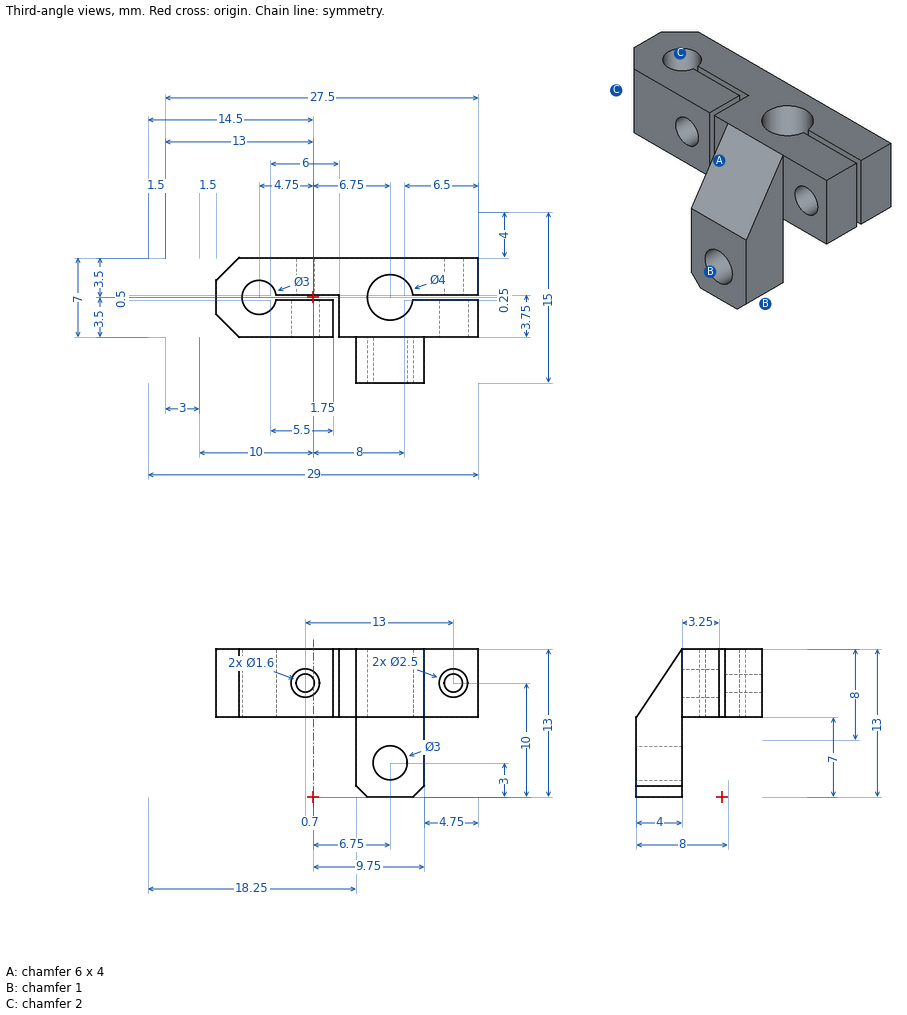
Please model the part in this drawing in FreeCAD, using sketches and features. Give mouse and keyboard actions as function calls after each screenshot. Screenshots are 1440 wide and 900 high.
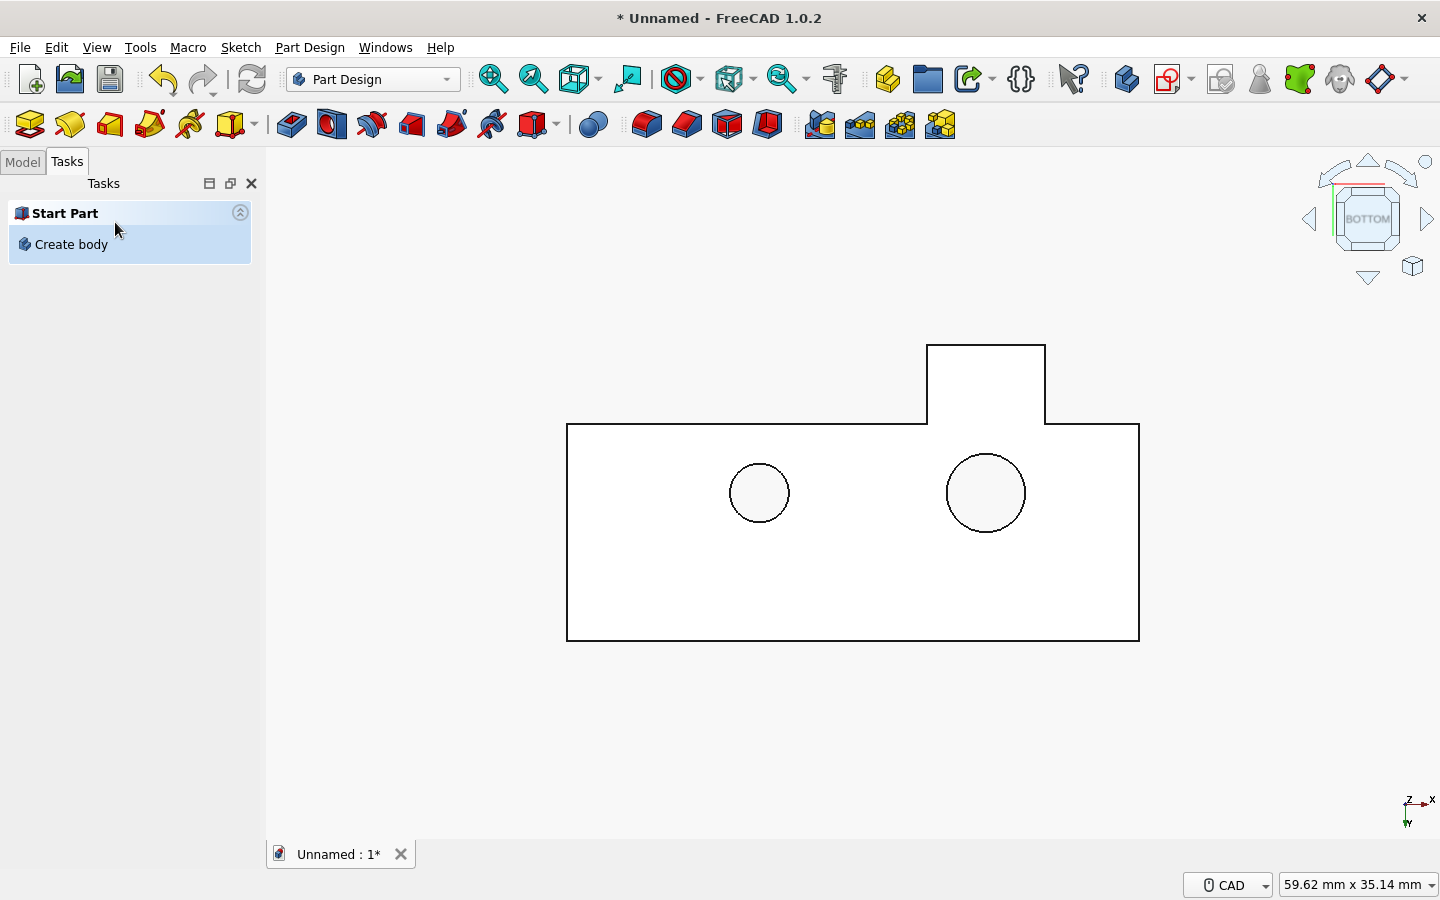
click(853, 534)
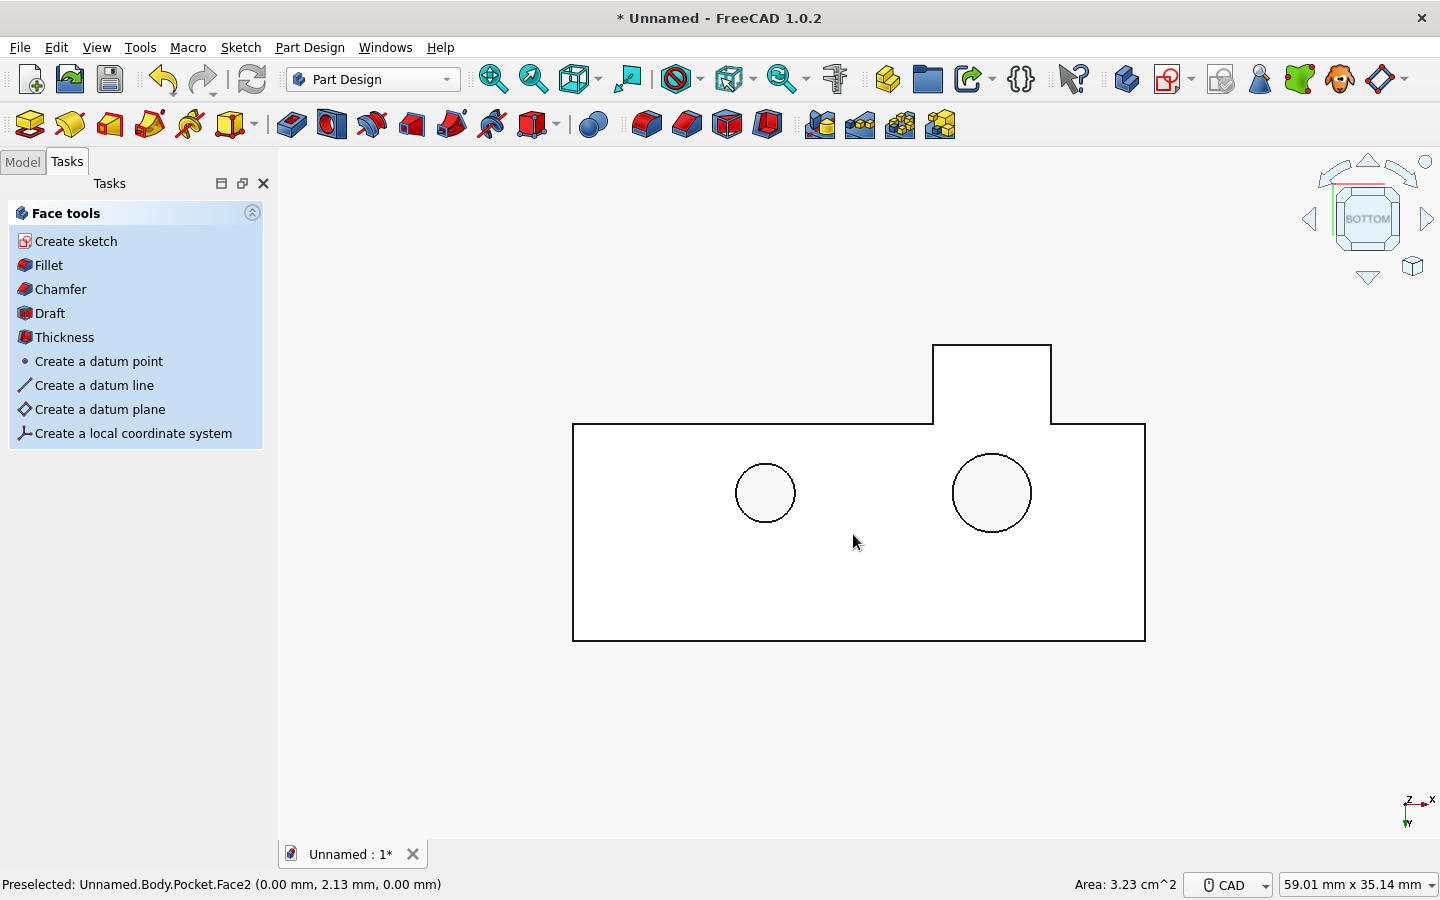
click(1168, 80)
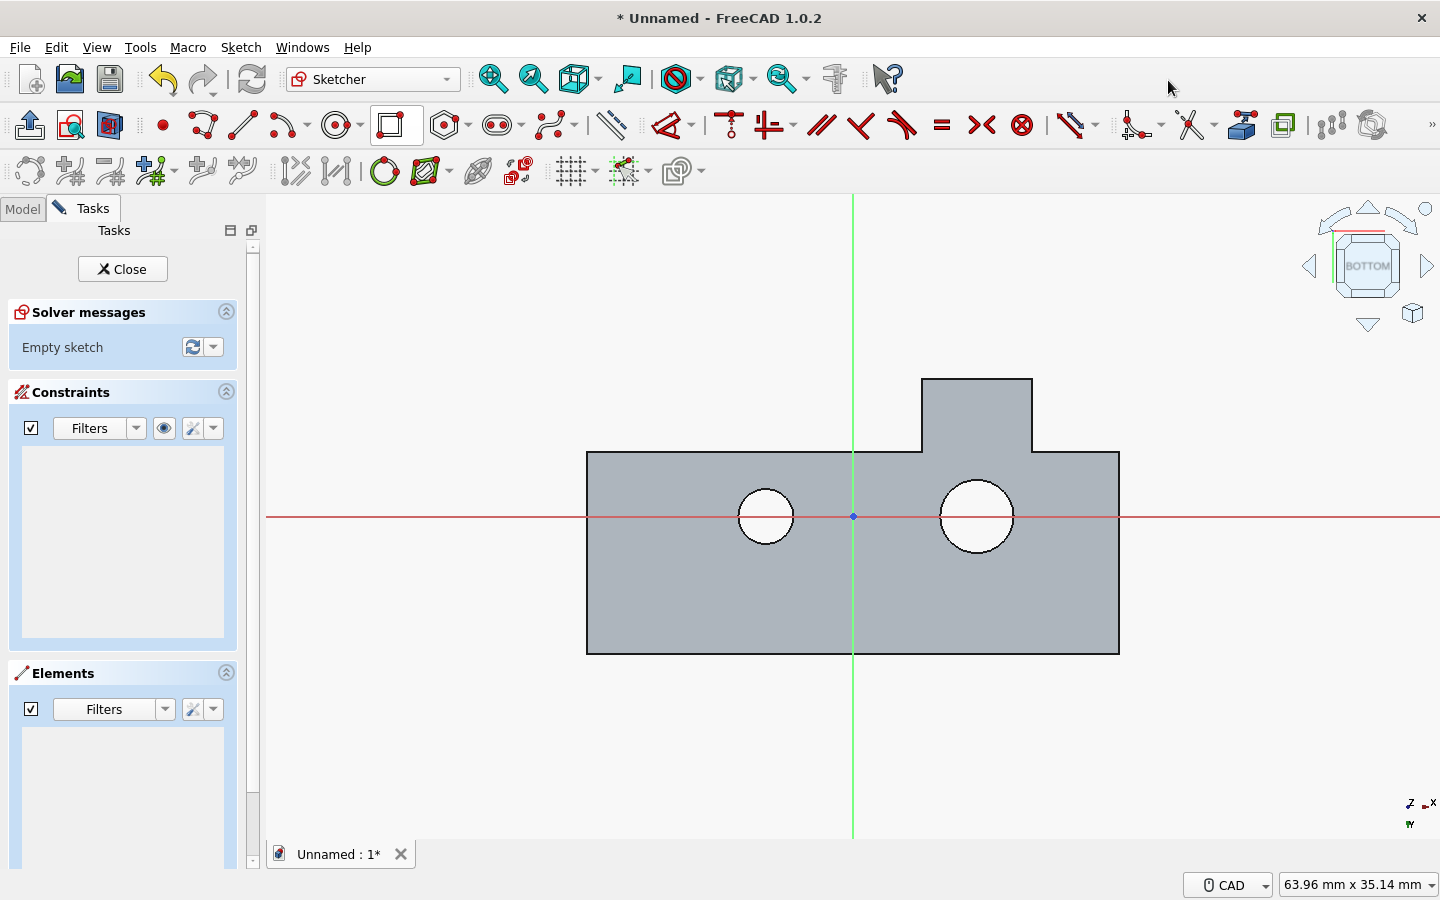
click(390, 126)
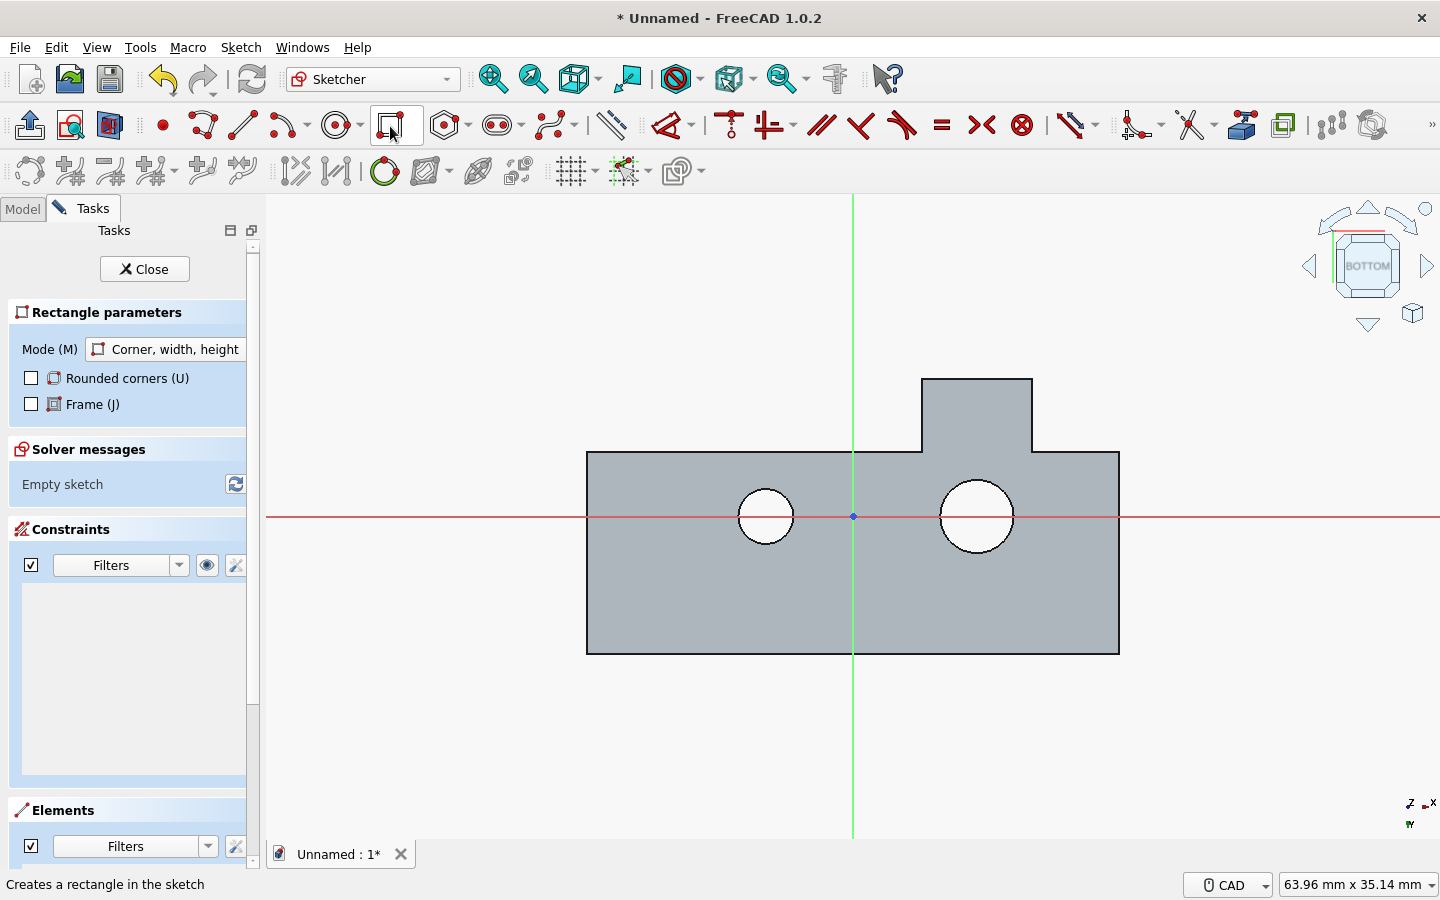
click(587, 581)
move(1119, 654)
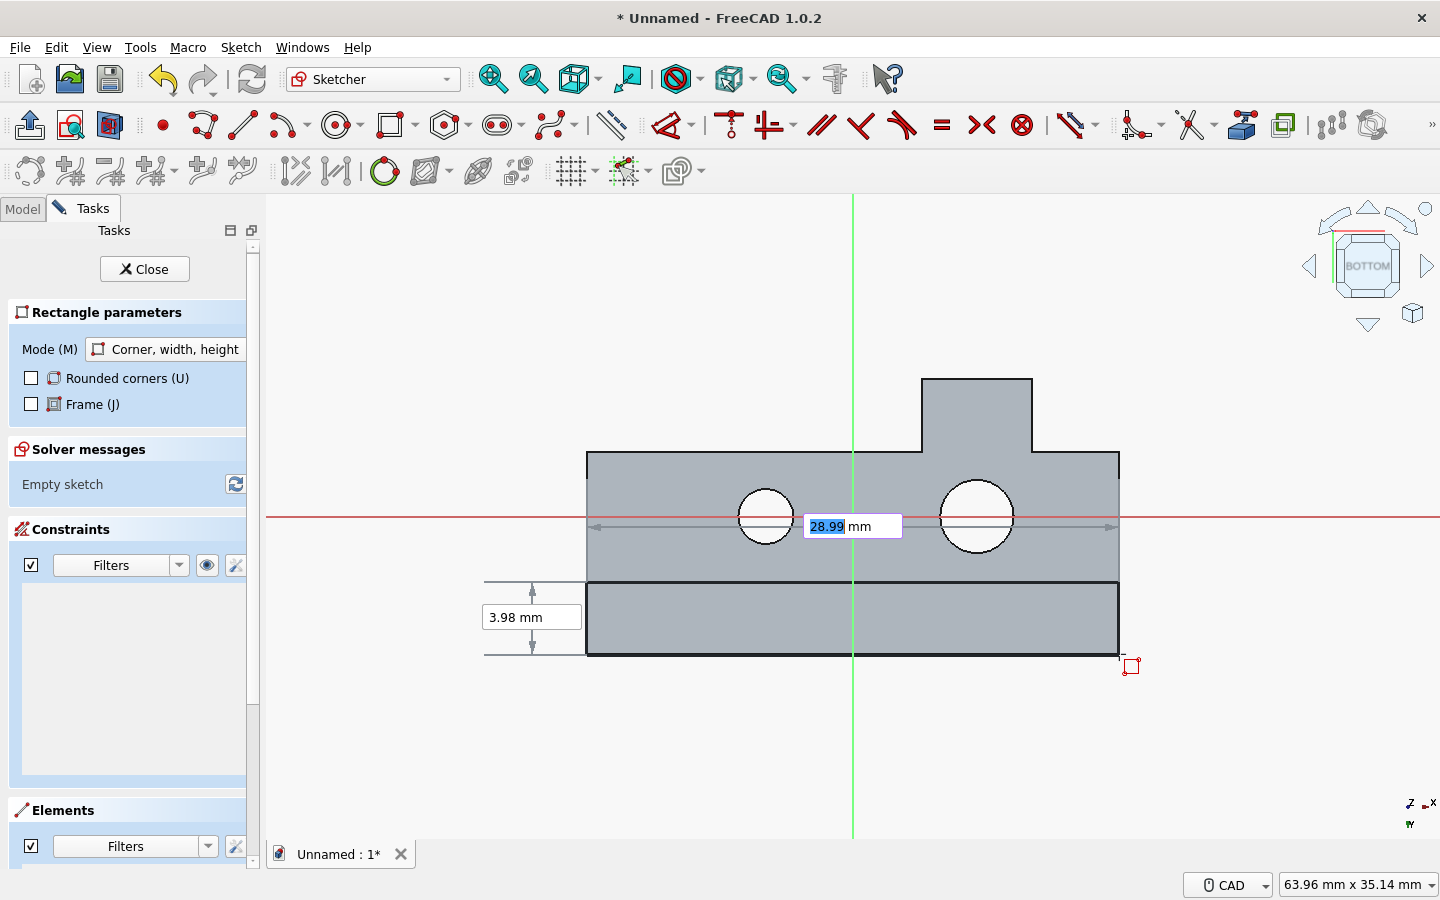
text(29)
key(Tab)
text(4)
key(Return)
key(Escape)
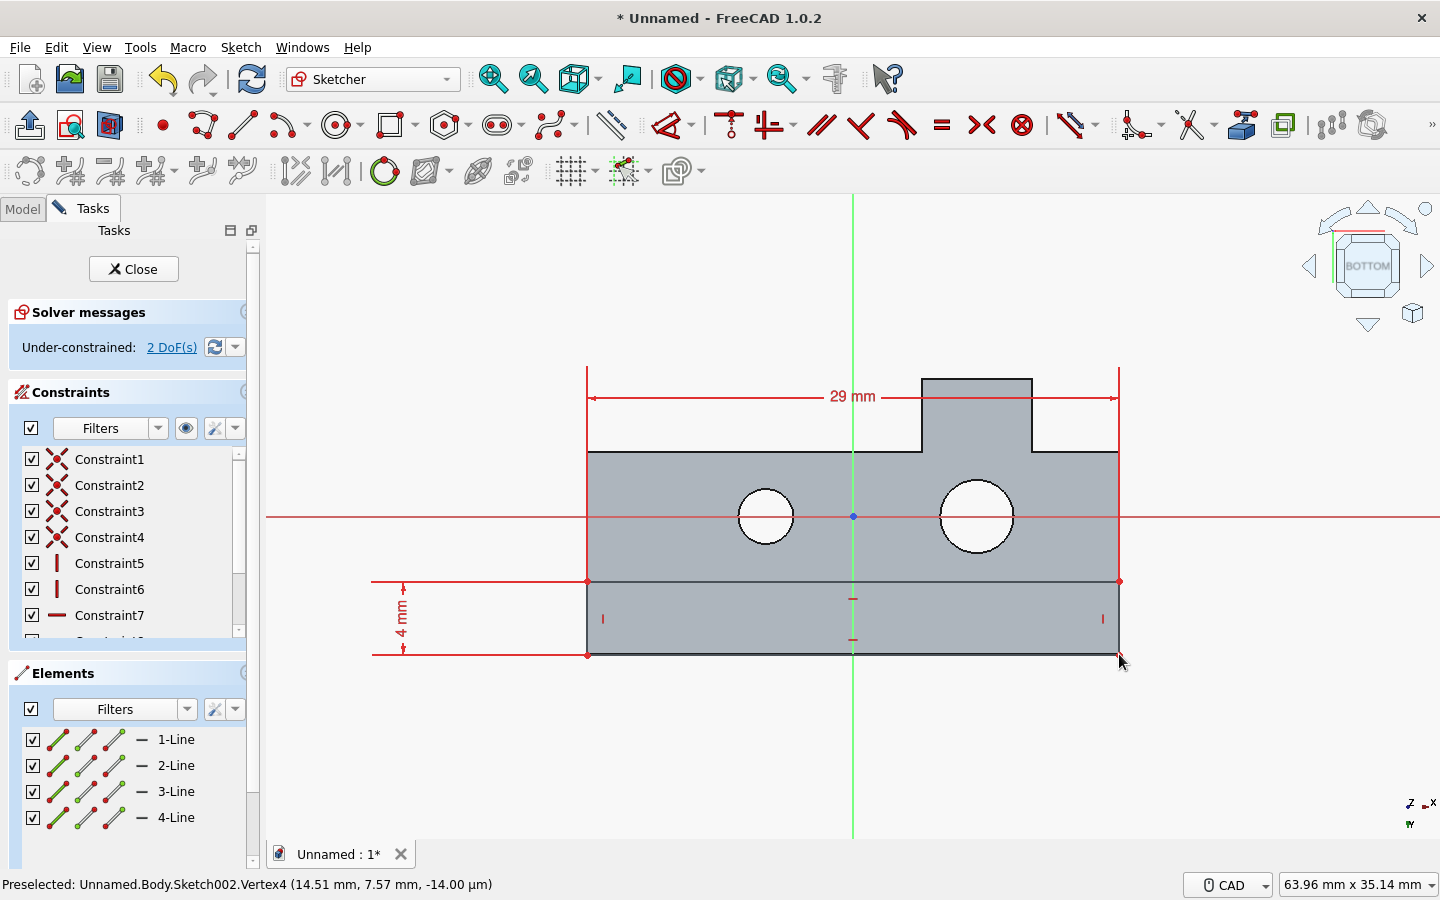
click(666, 126)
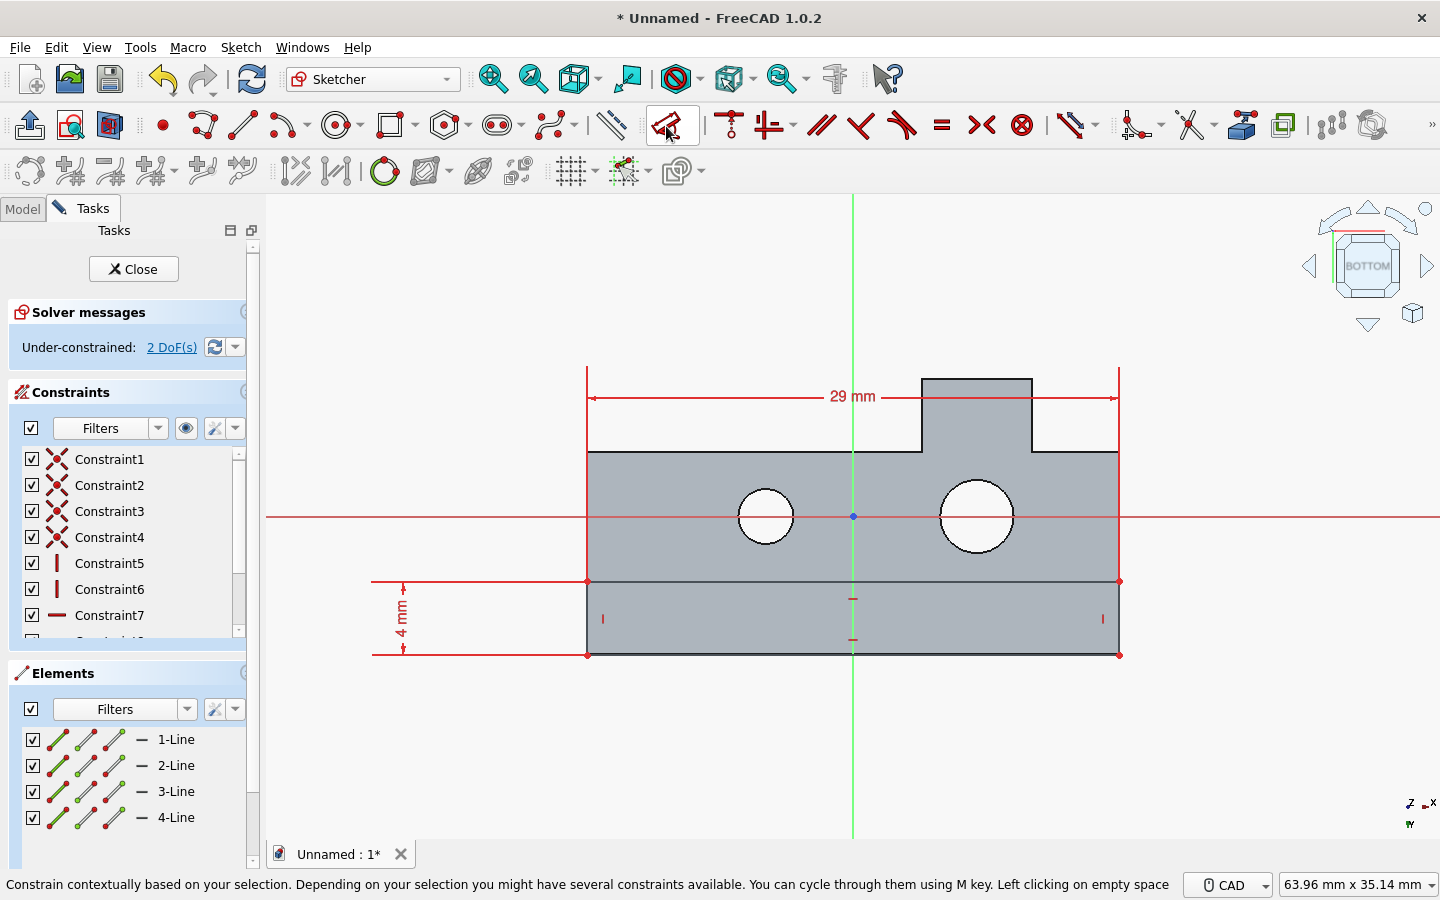
click(587, 582)
click(553, 549)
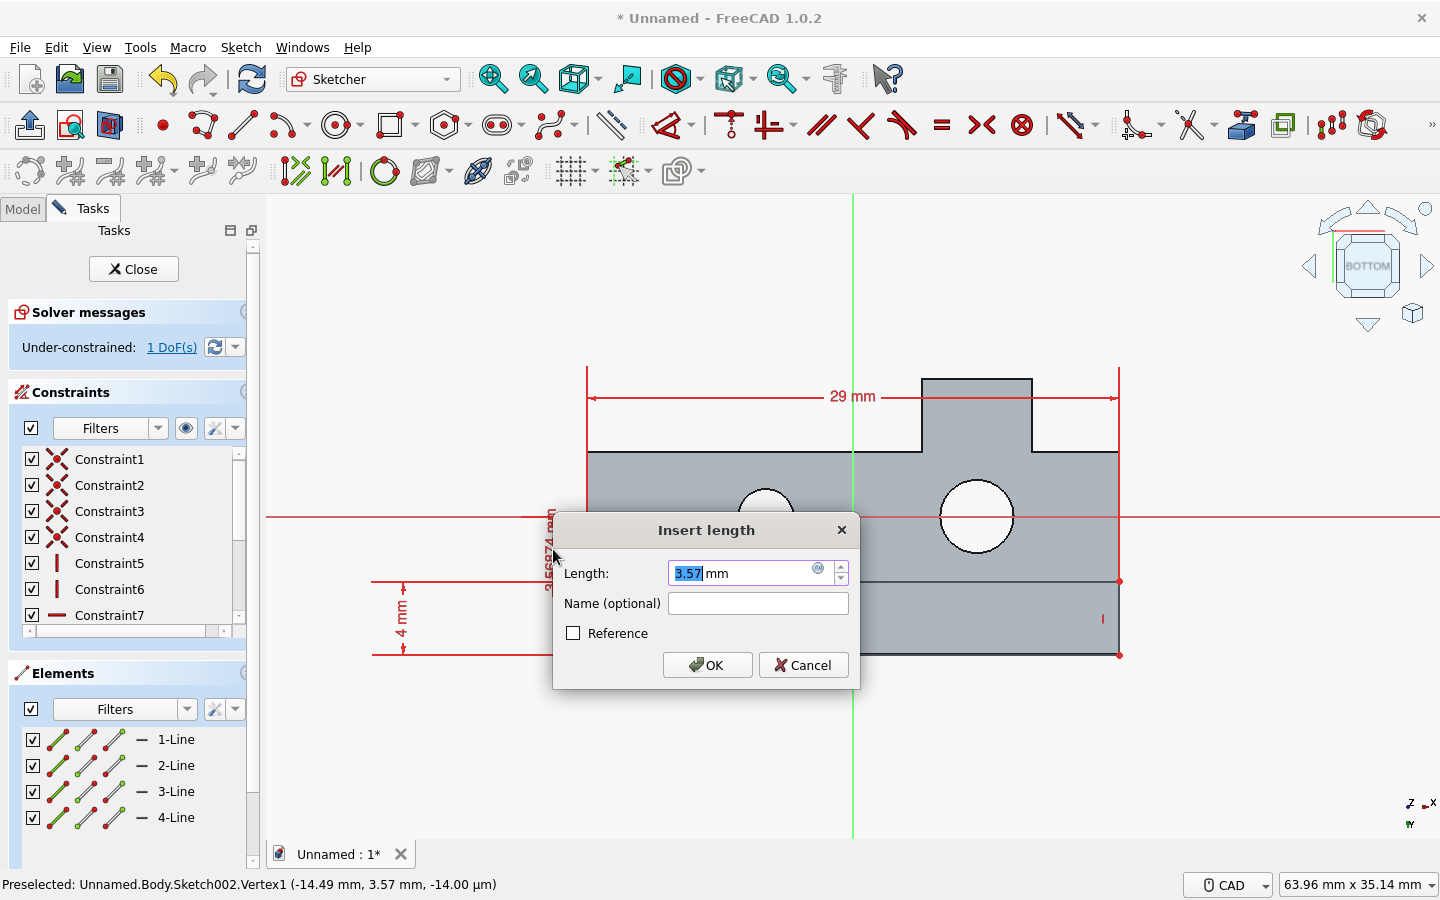
text(3.5)
key(Return)